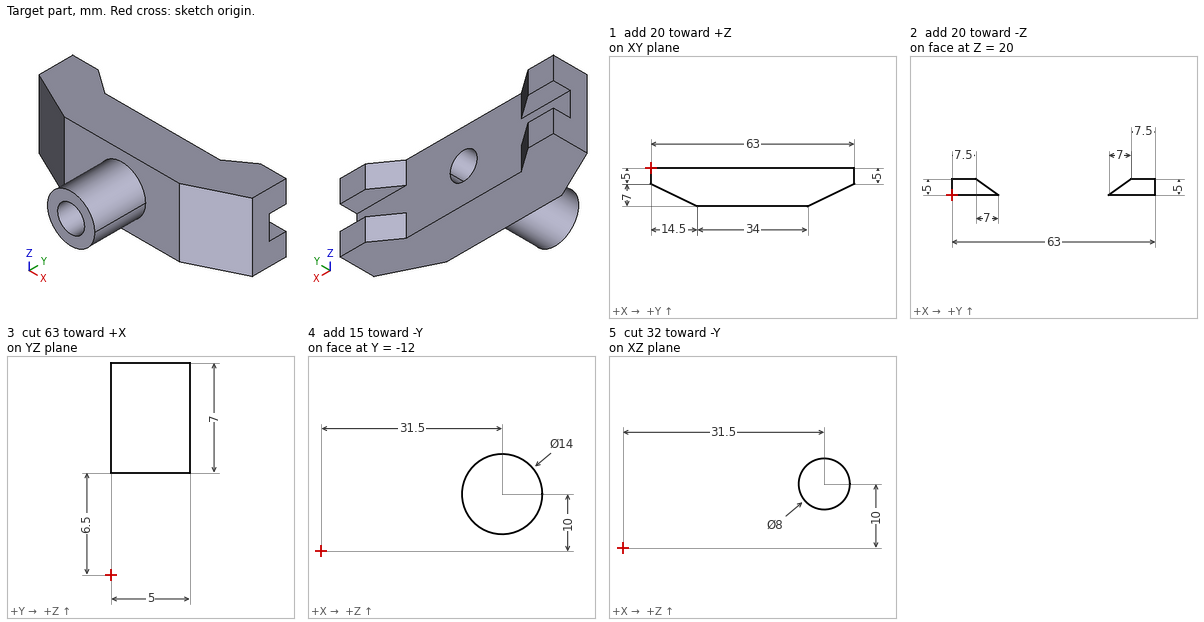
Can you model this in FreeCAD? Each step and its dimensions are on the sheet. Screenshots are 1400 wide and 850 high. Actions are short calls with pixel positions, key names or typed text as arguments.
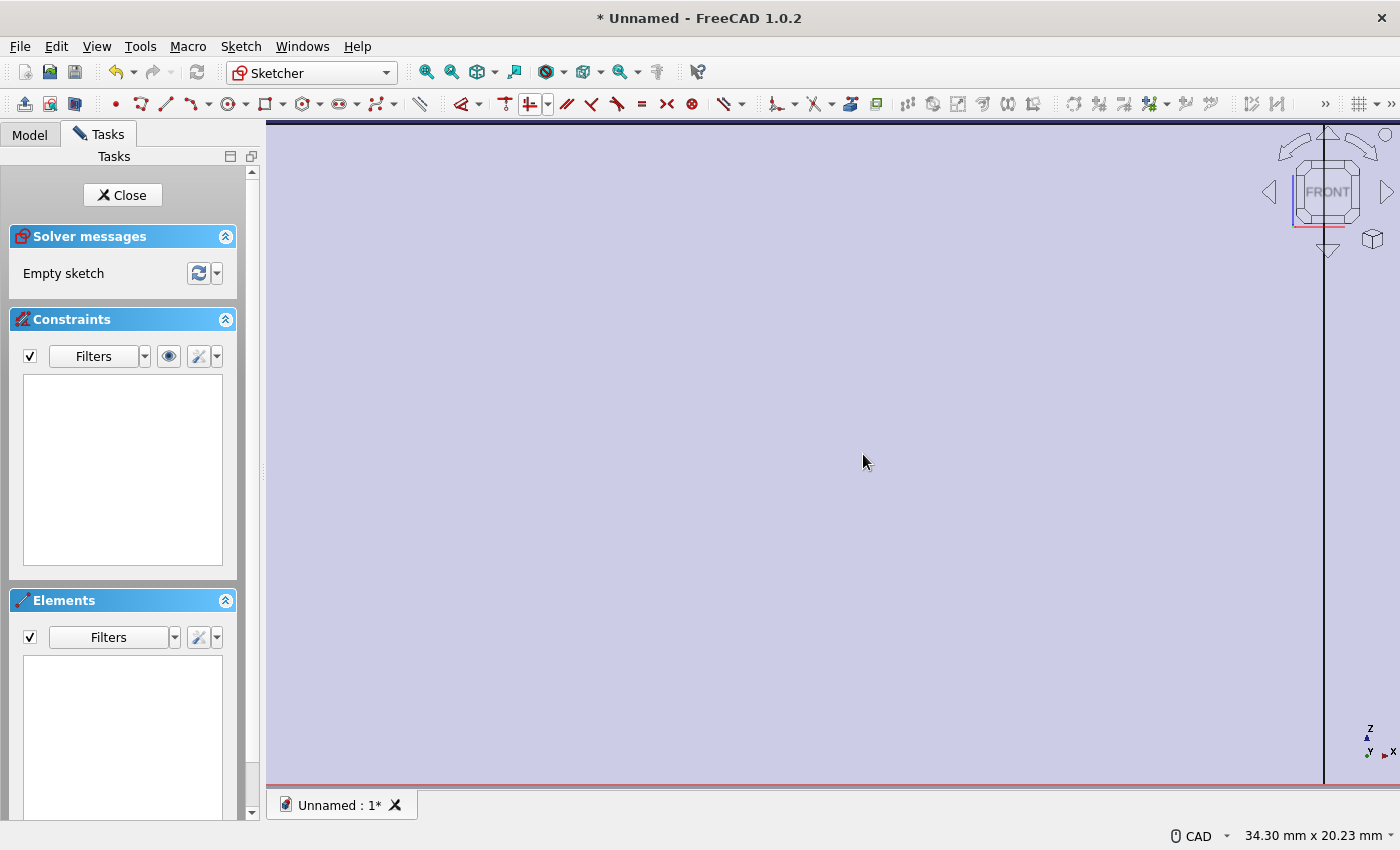
click(228, 104)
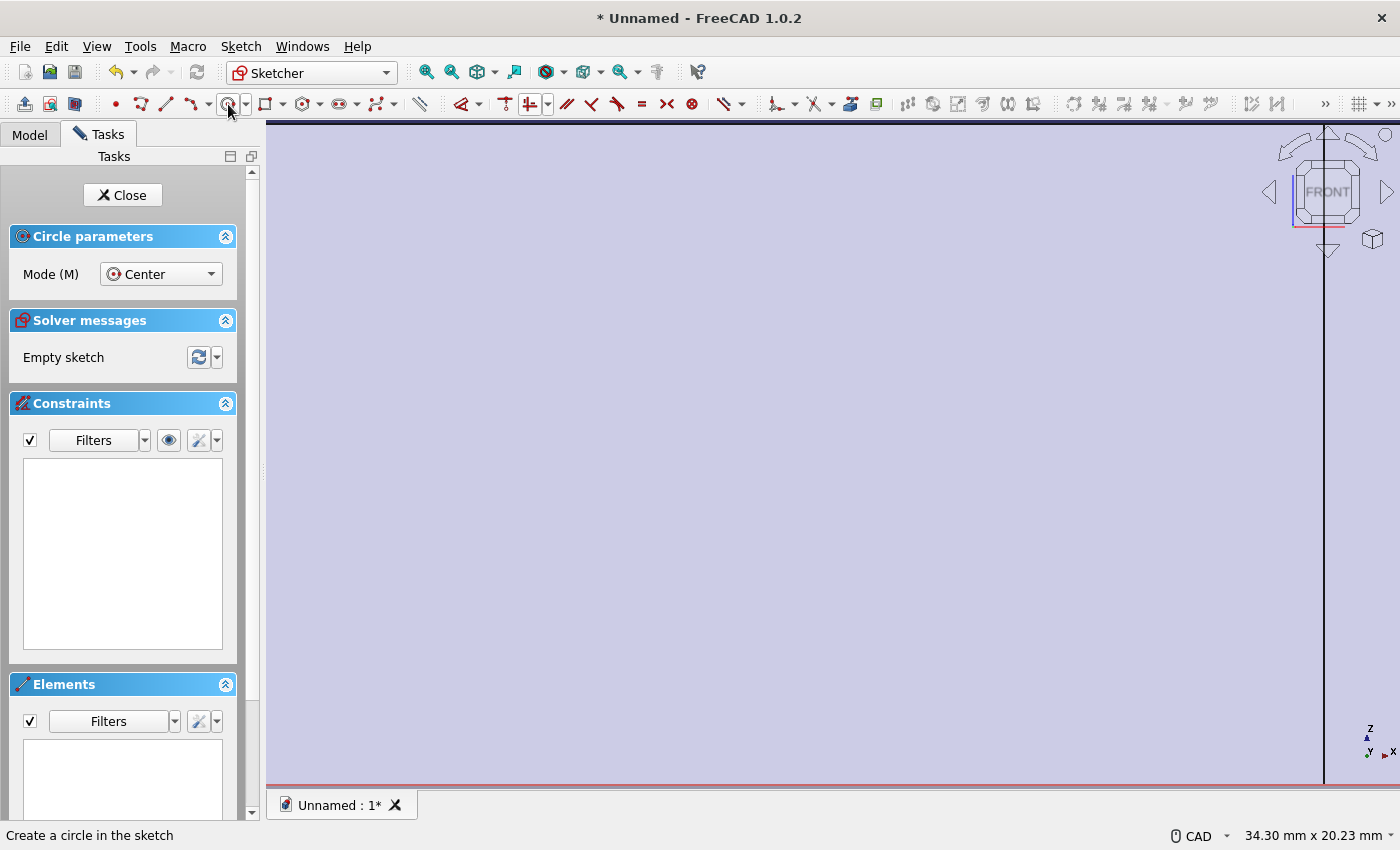
click(762, 454)
move(926, 291)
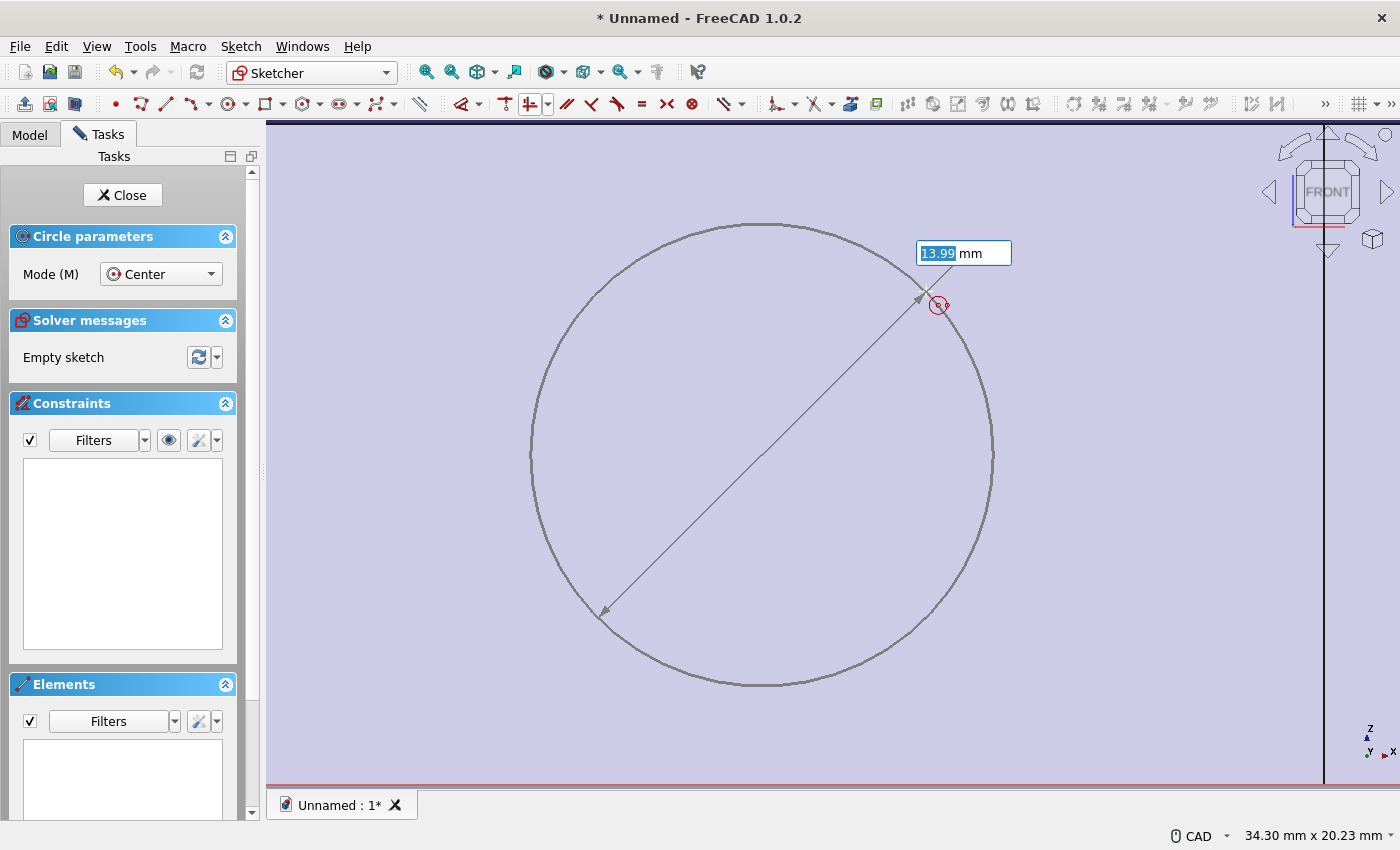
text(14)
key(Return)
key(Escape)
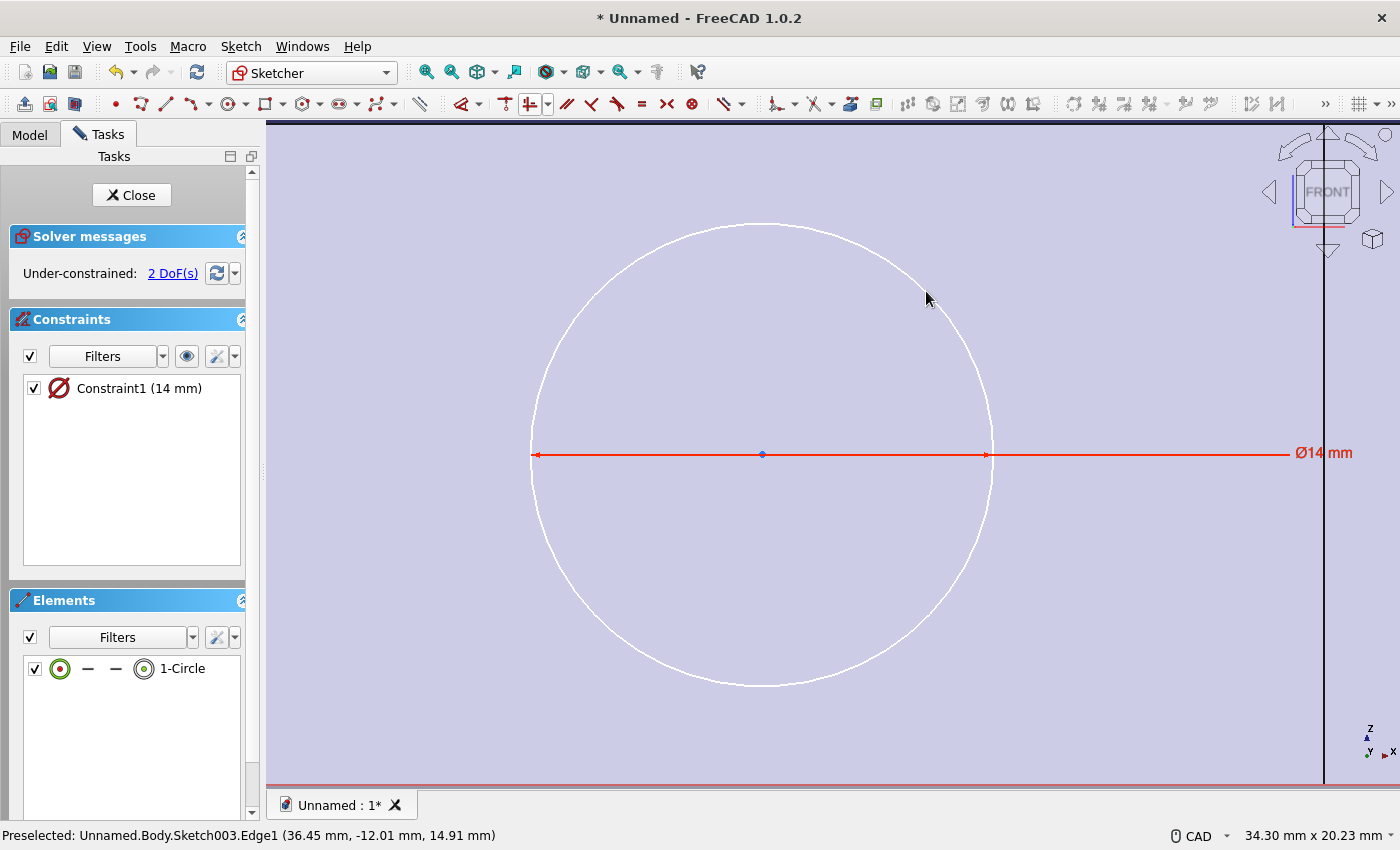
click(460, 104)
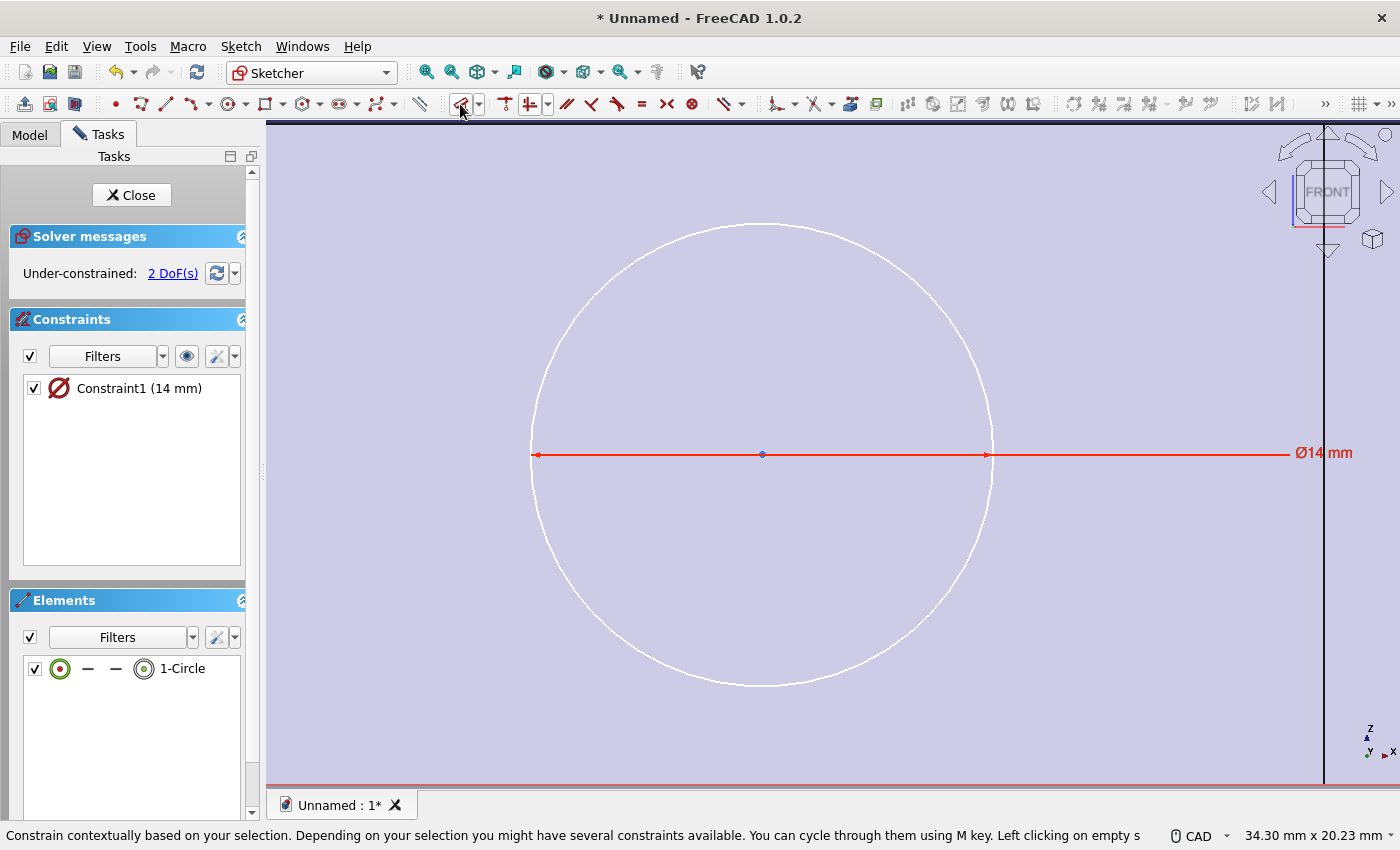
click(762, 455)
click(796, 608)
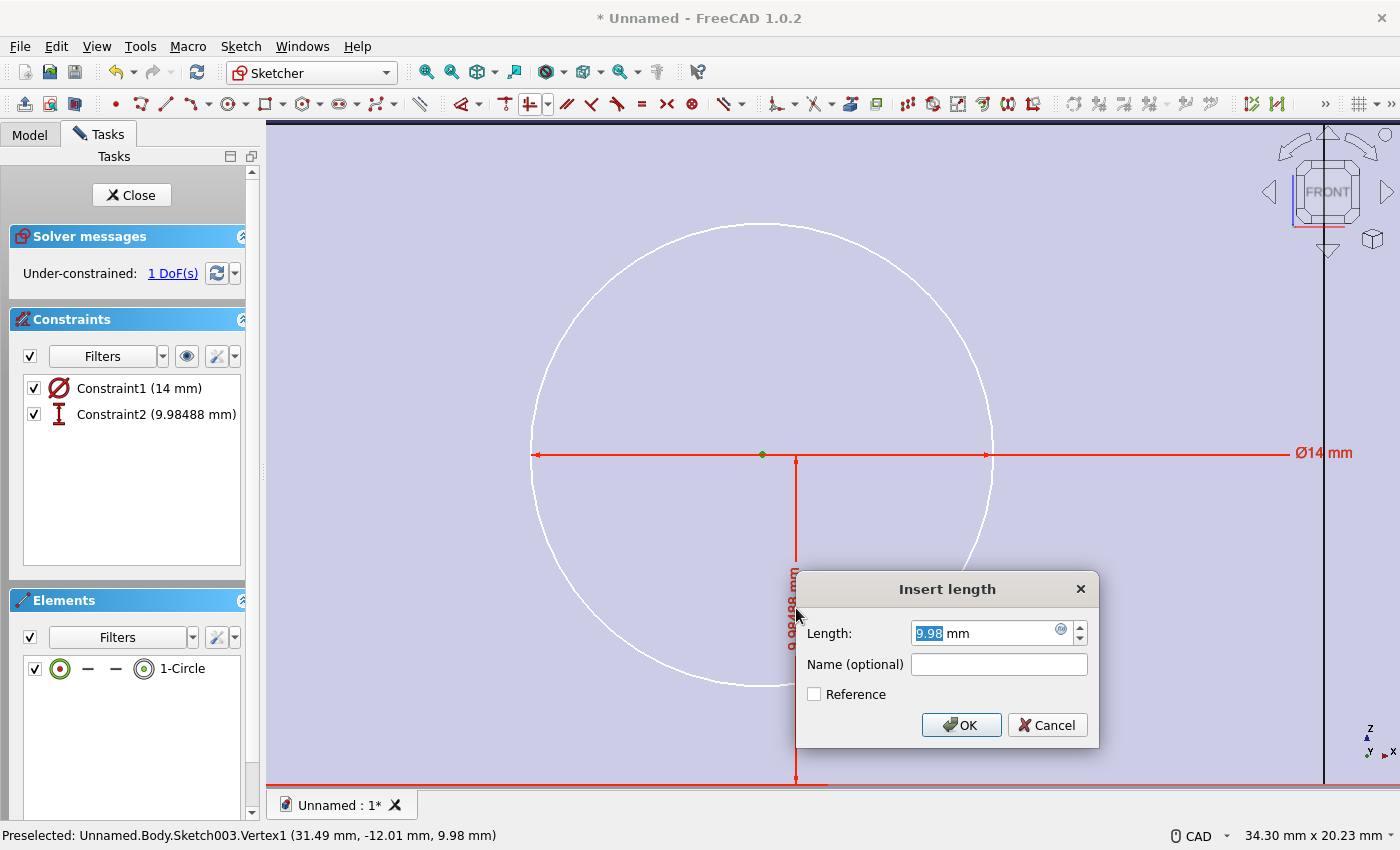
text(10)
key(Return)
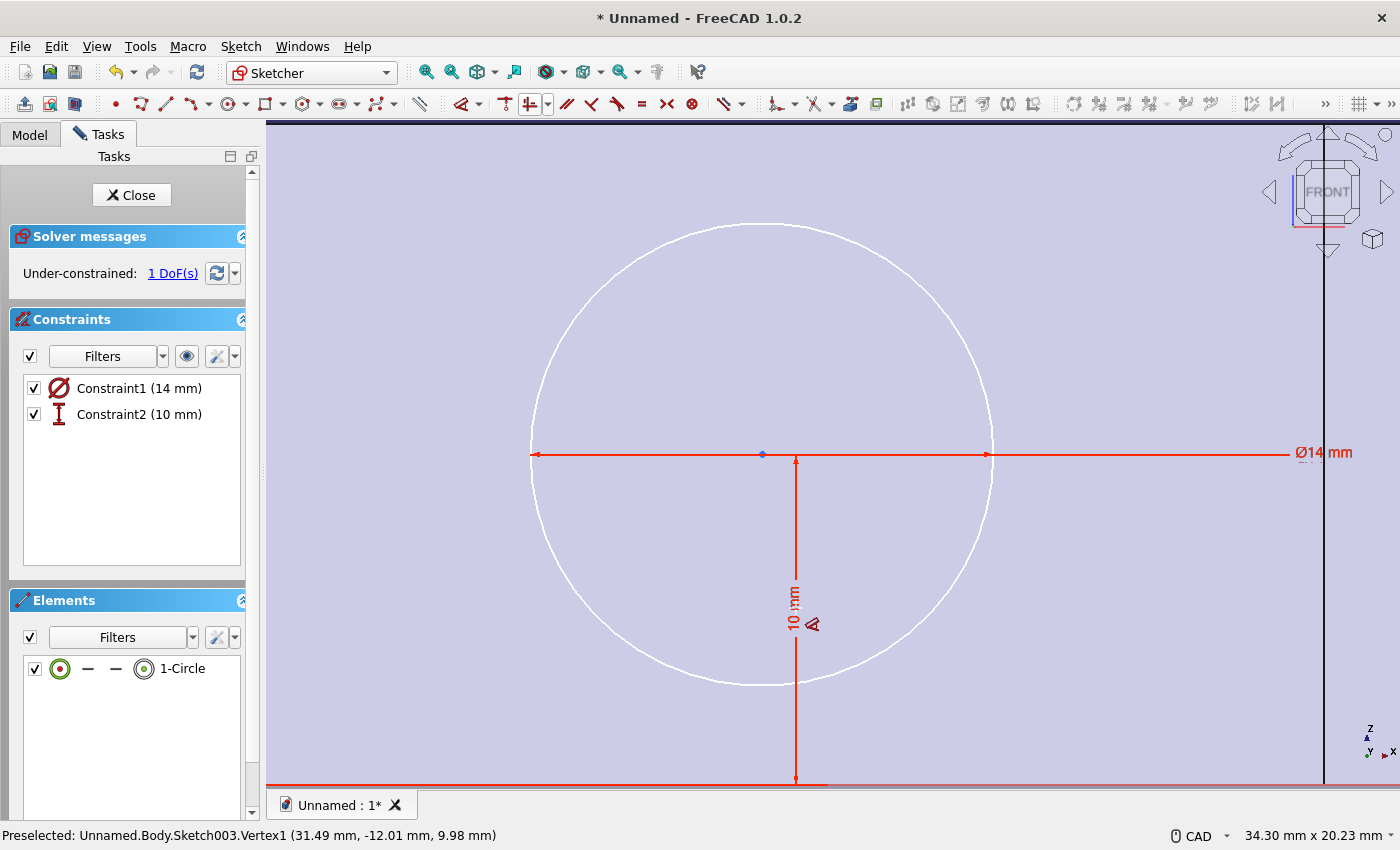
click(762, 454)
click(420, 420)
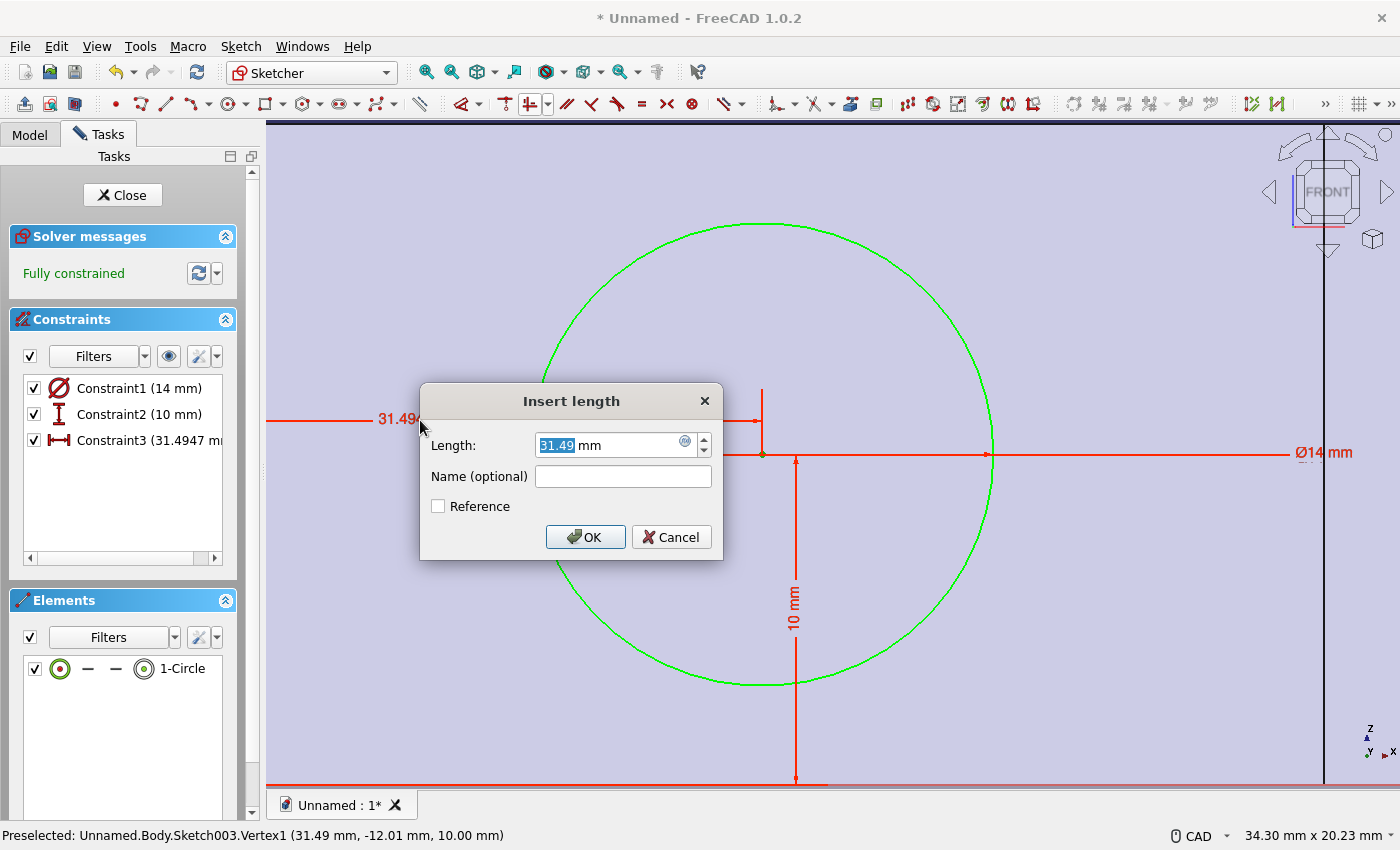
text(31.5)
key(Return)
key(Escape)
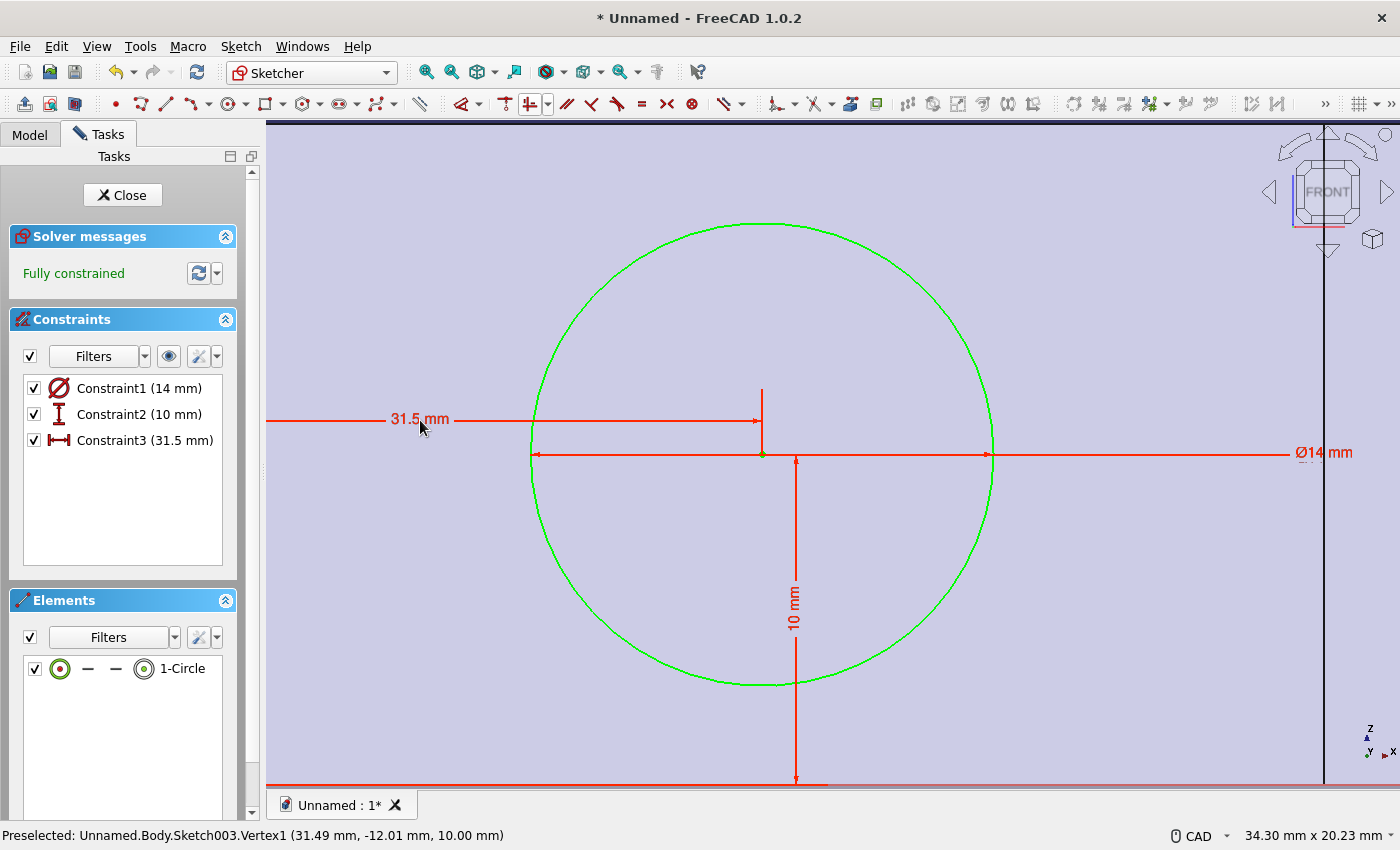
click(123, 195)